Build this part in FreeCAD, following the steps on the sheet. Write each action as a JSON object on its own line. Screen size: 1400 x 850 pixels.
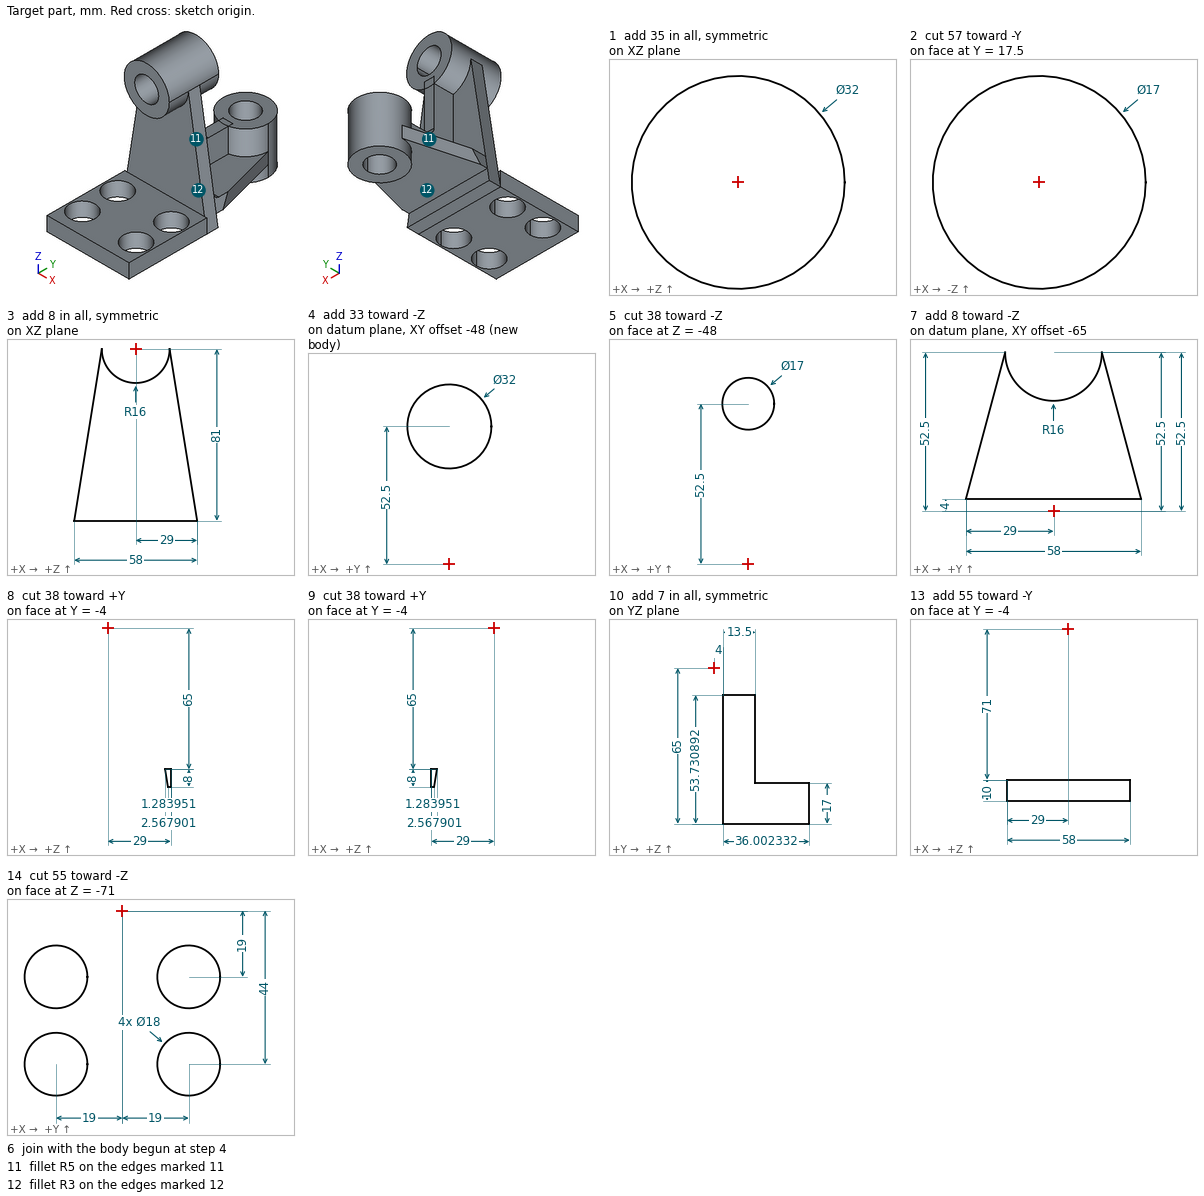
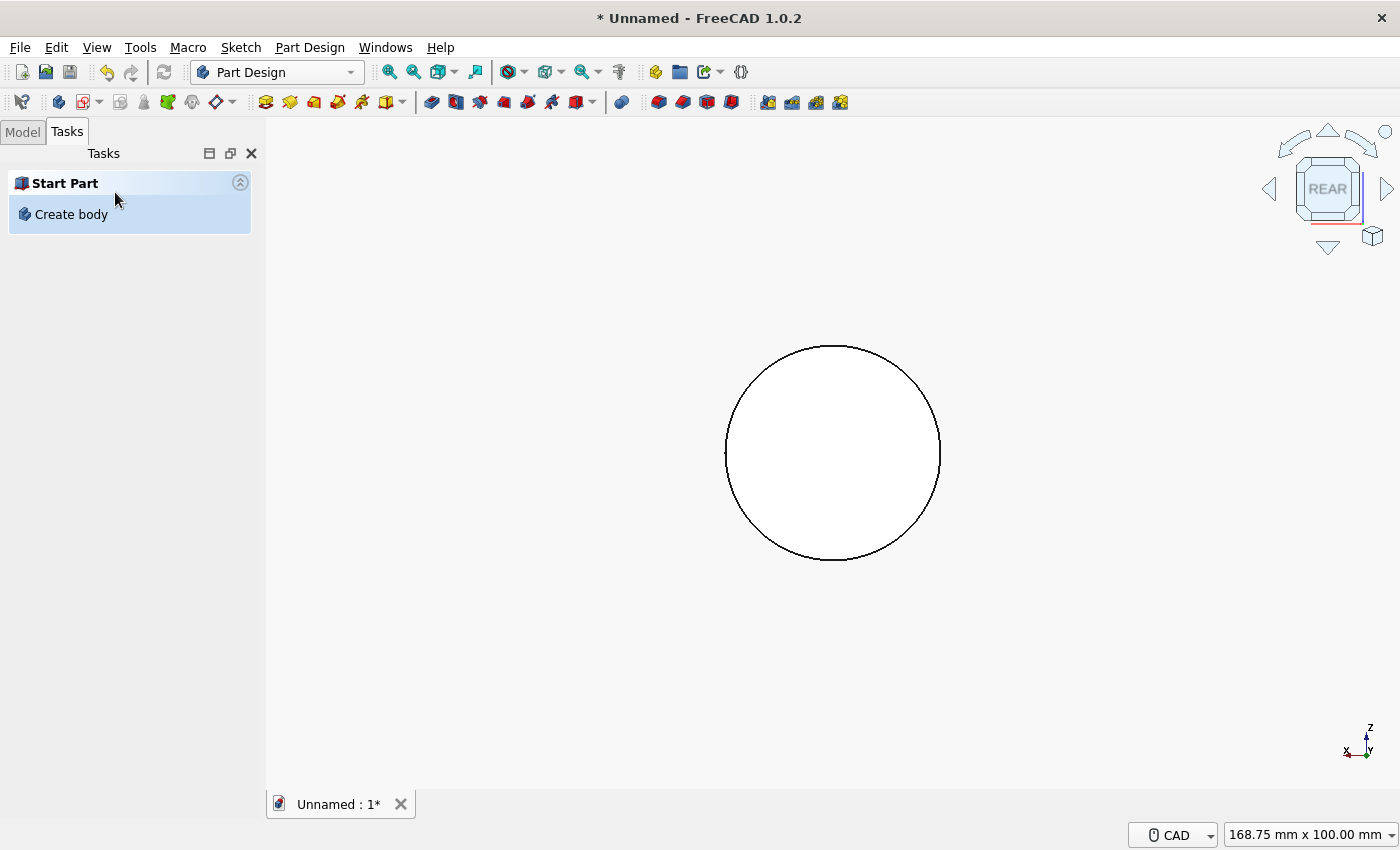
{"action": "left_click", "coordinate": [390, 72]}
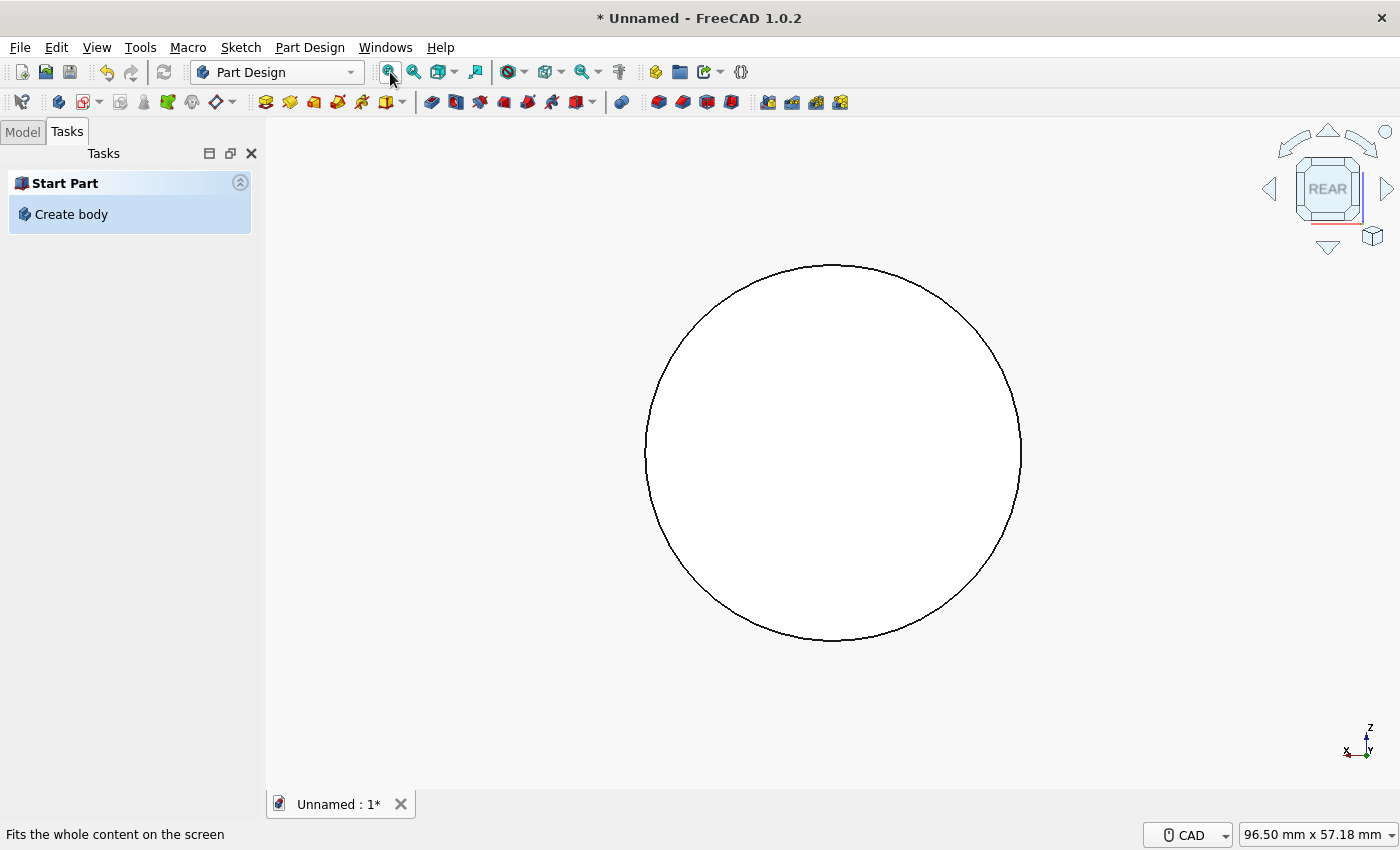
{"action": "left_click", "coordinate": [833, 452]}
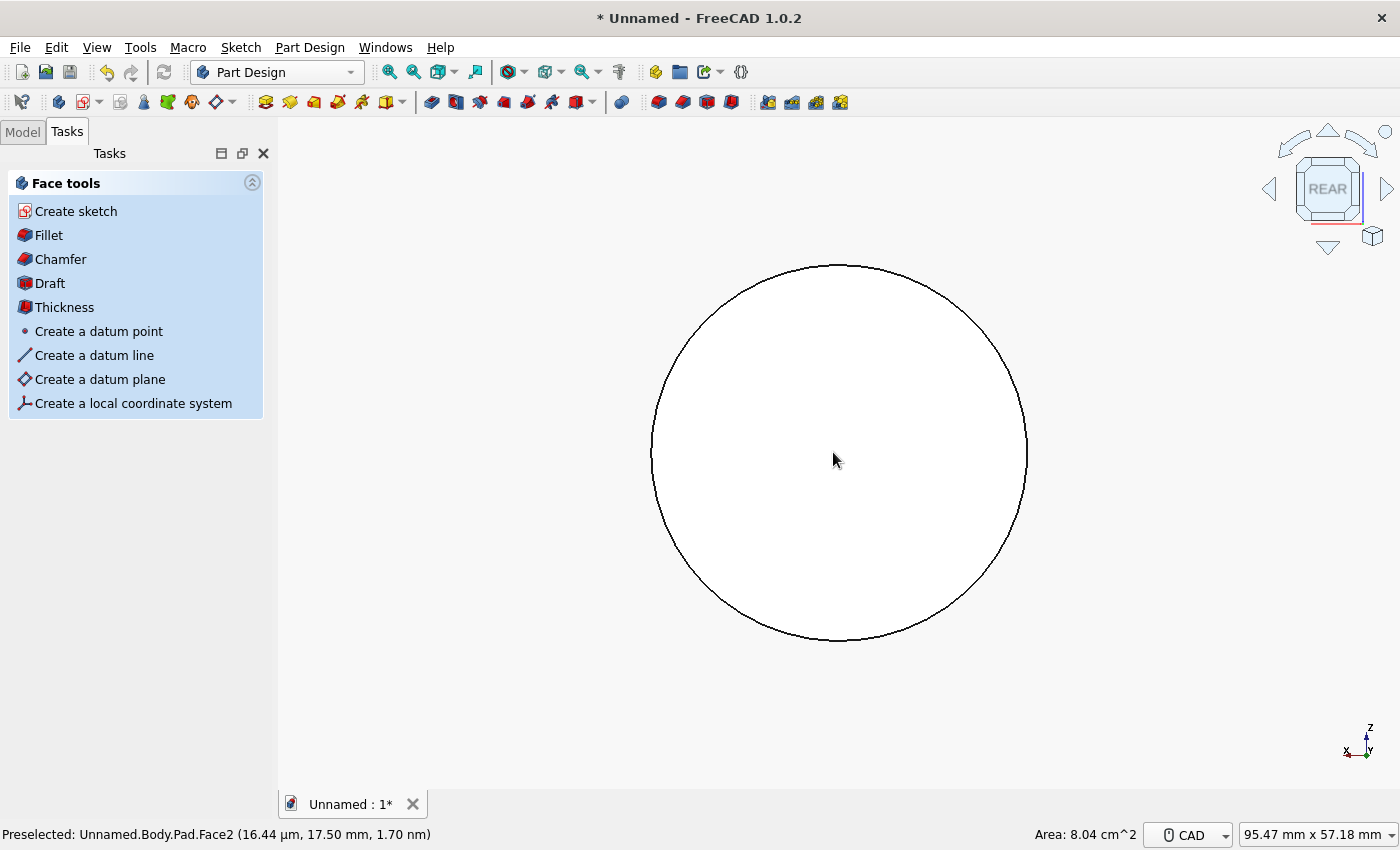
{"action": "left_click", "coordinate": [84, 102]}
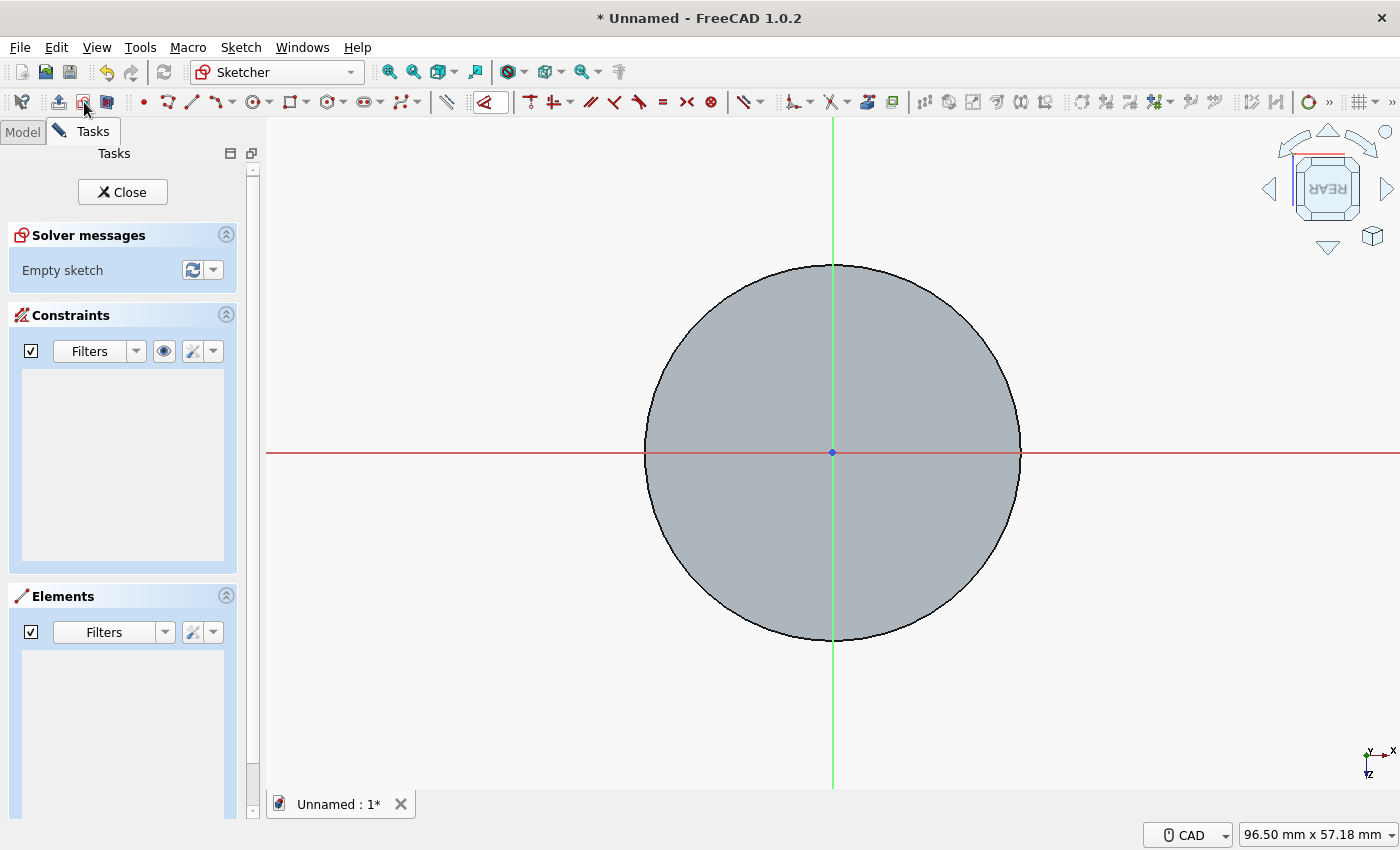
{"action": "scroll", "coordinate": [889, 453], "scroll_direction": "up", "scroll_amount": 4}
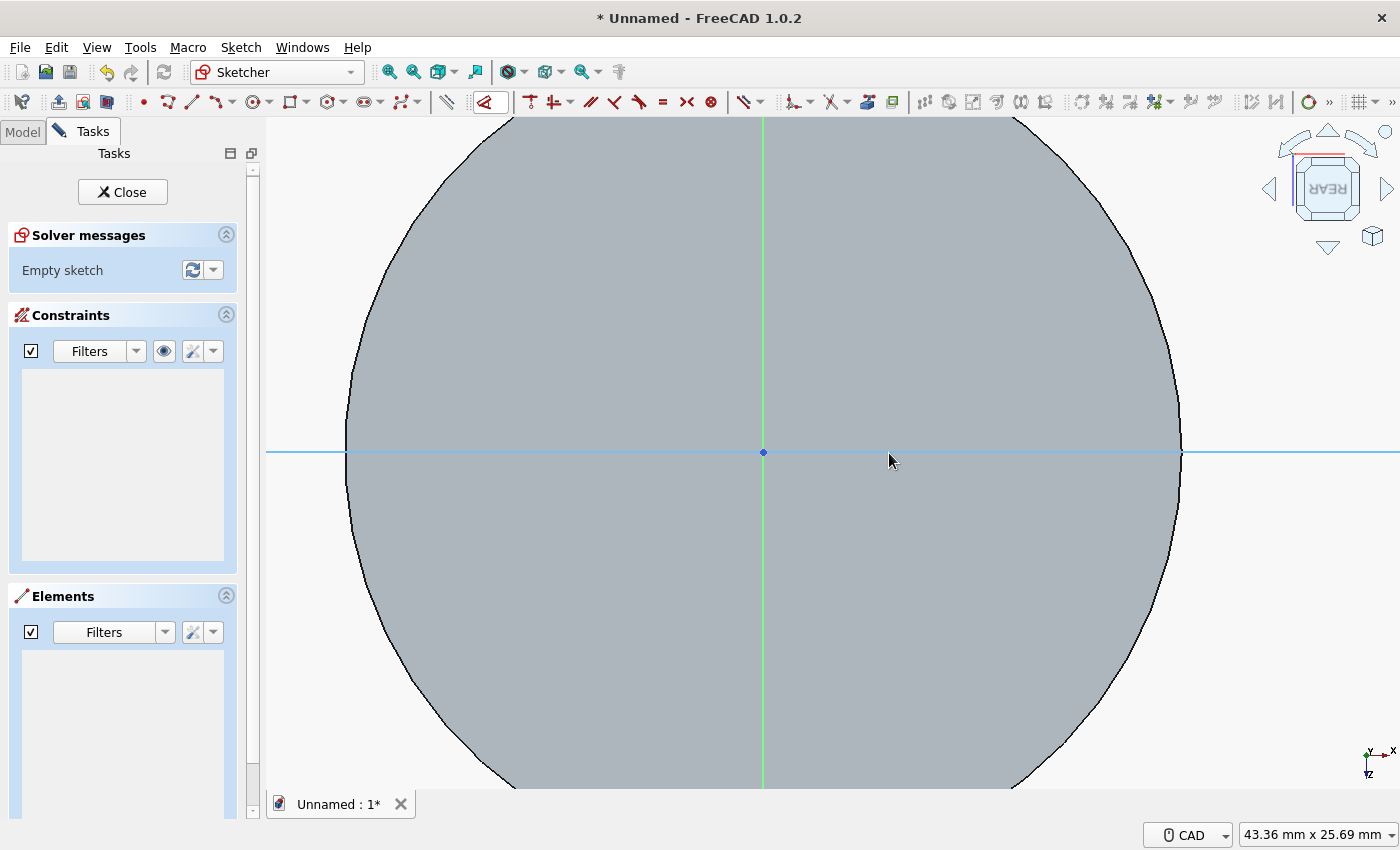
{"action": "key", "text": "g c"}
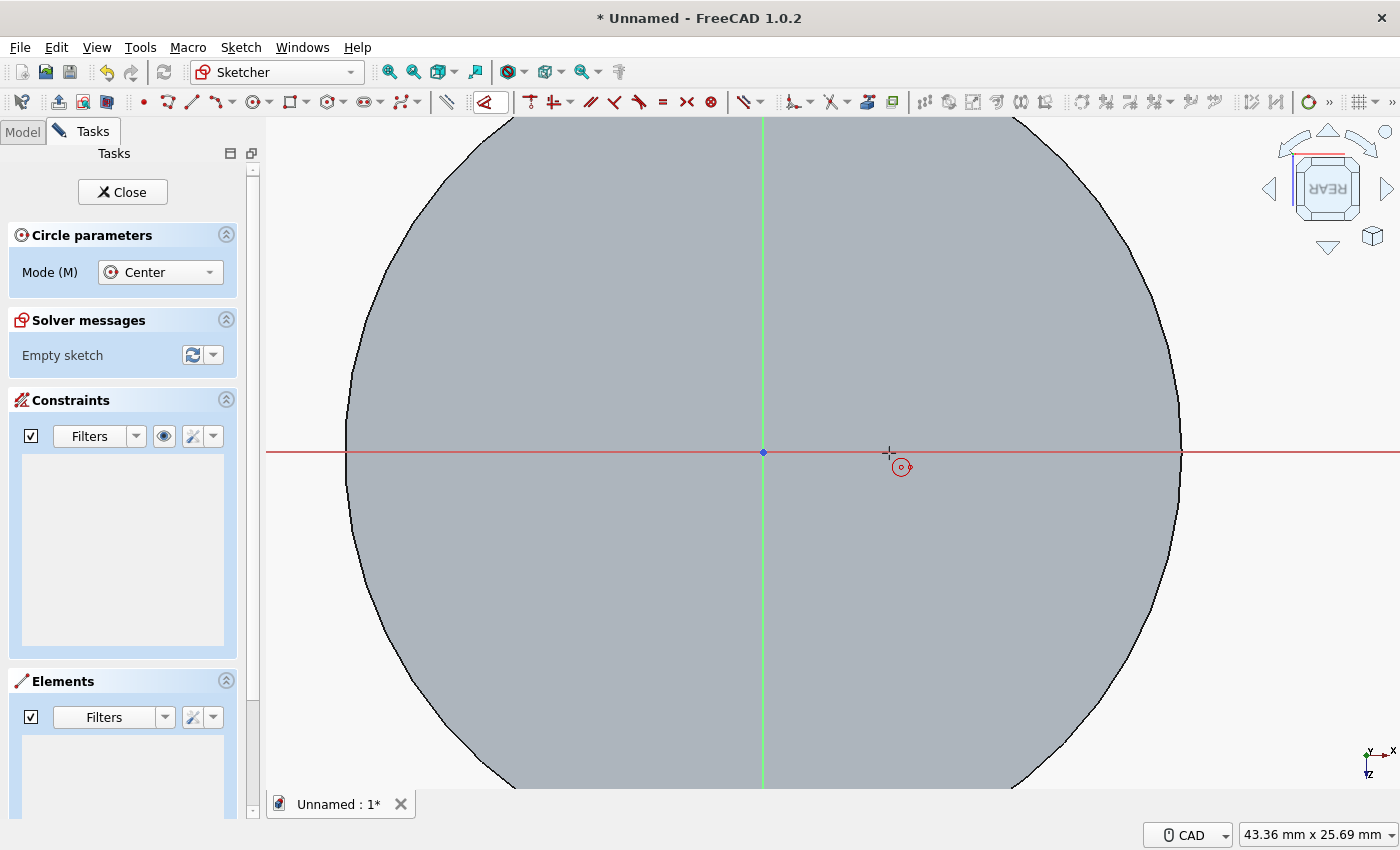
{"action": "left_click", "coordinate": [763, 452]}
{"action": "left_click", "coordinate": [920, 295]}
{"action": "key", "text": "Escape"}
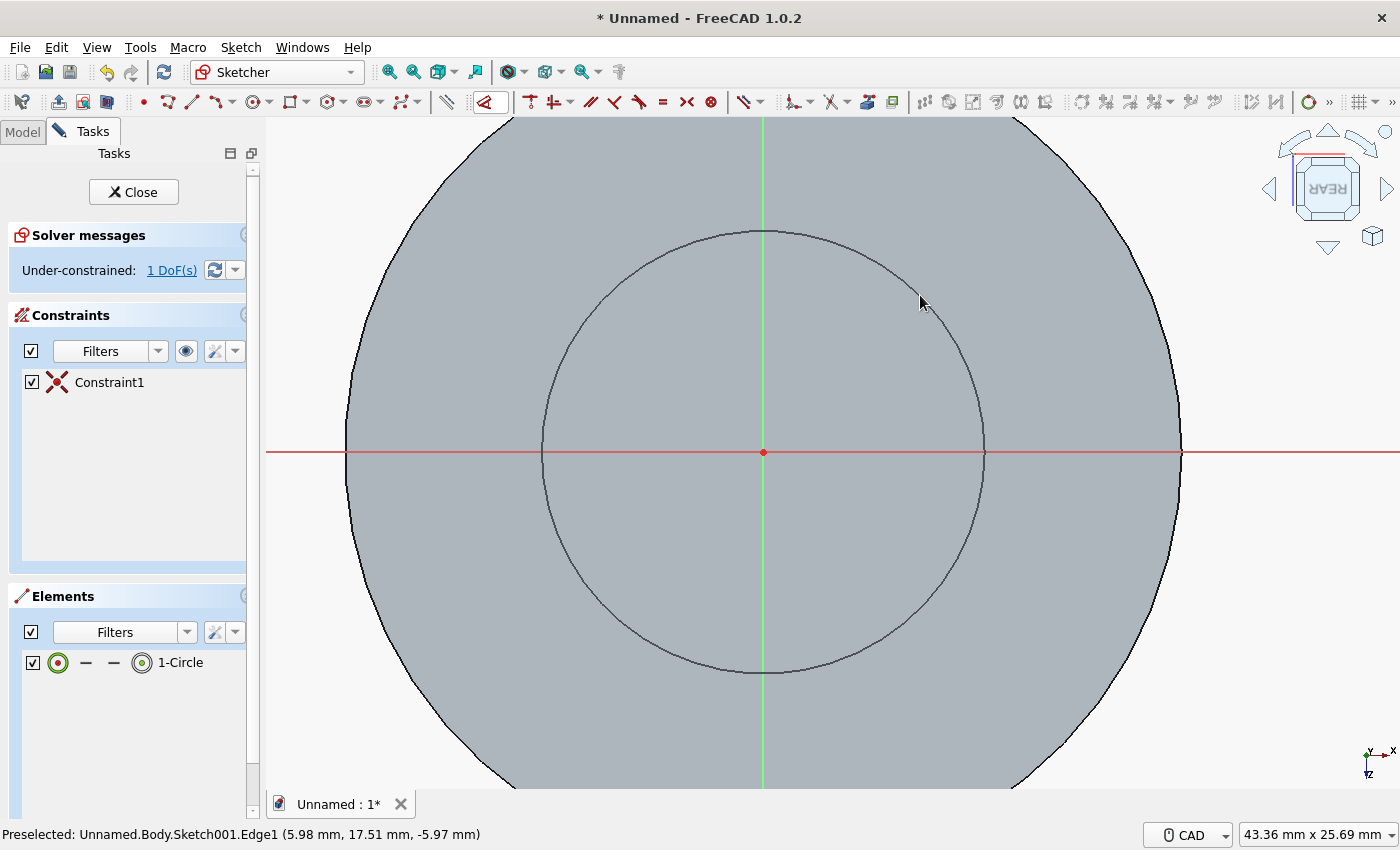
{"action": "key", "text": "d"}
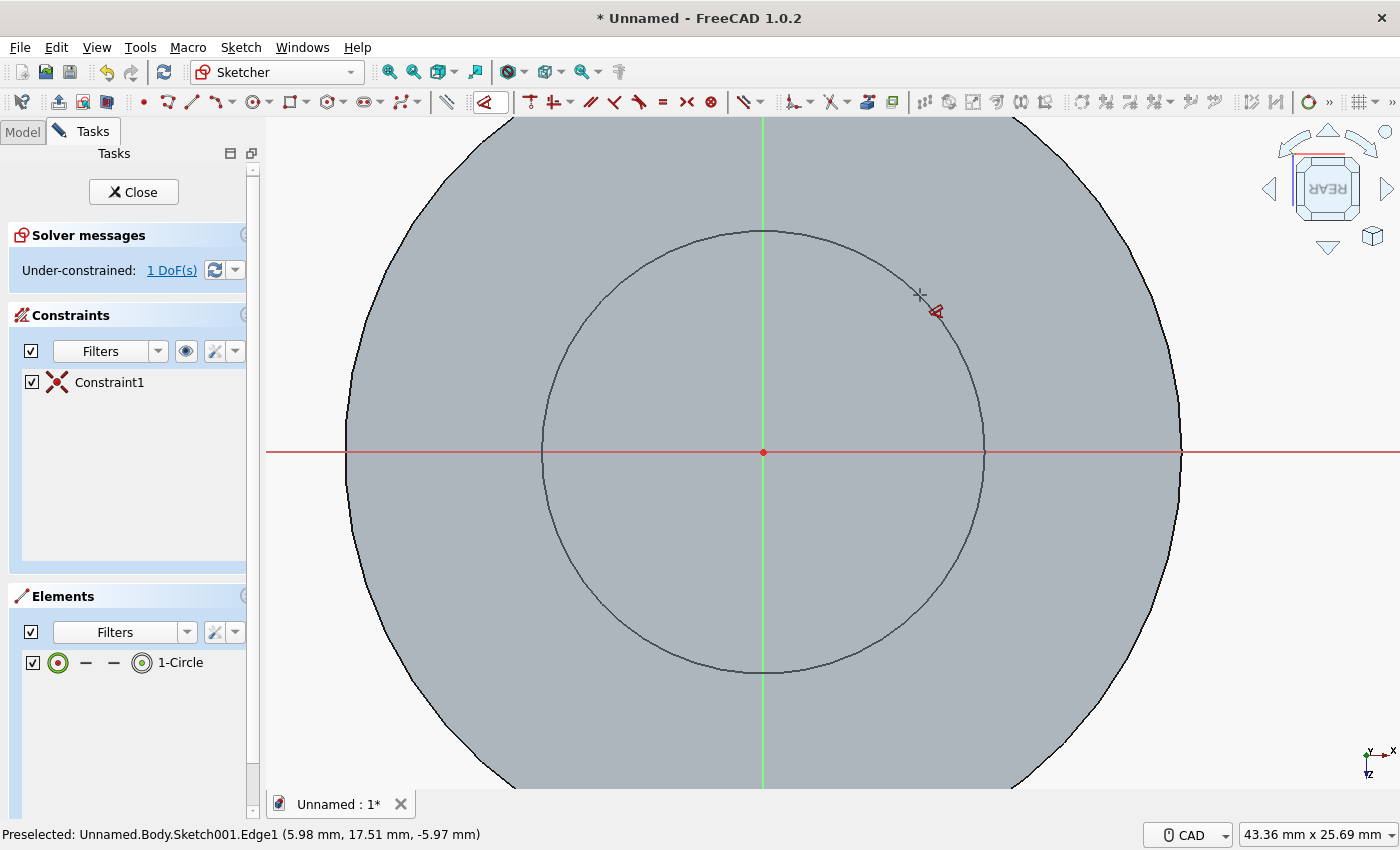
{"action": "left_click", "coordinate": [919, 295]}
{"action": "left_click", "coordinate": [942, 272]}